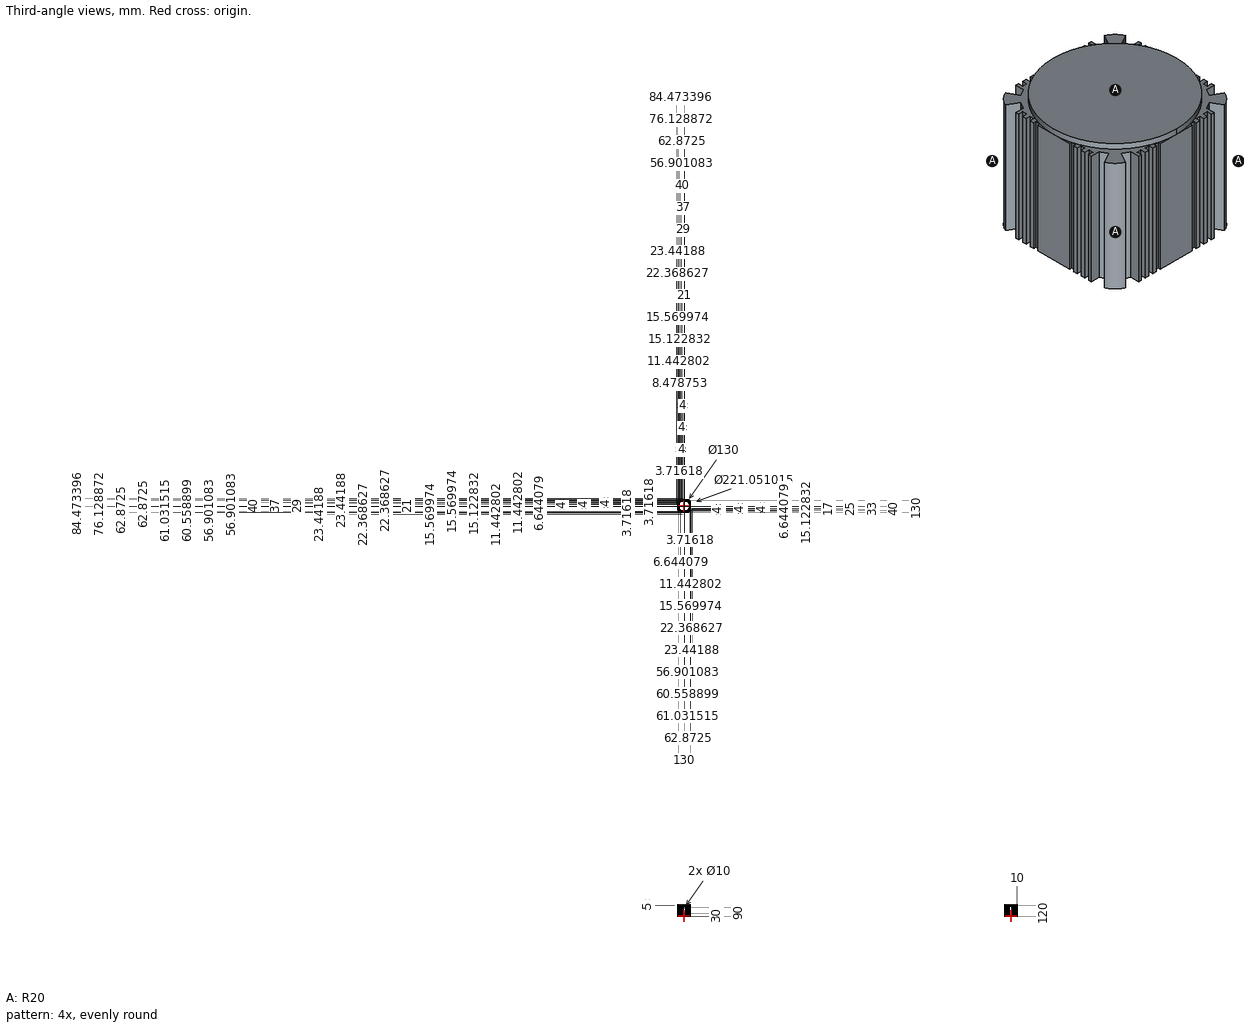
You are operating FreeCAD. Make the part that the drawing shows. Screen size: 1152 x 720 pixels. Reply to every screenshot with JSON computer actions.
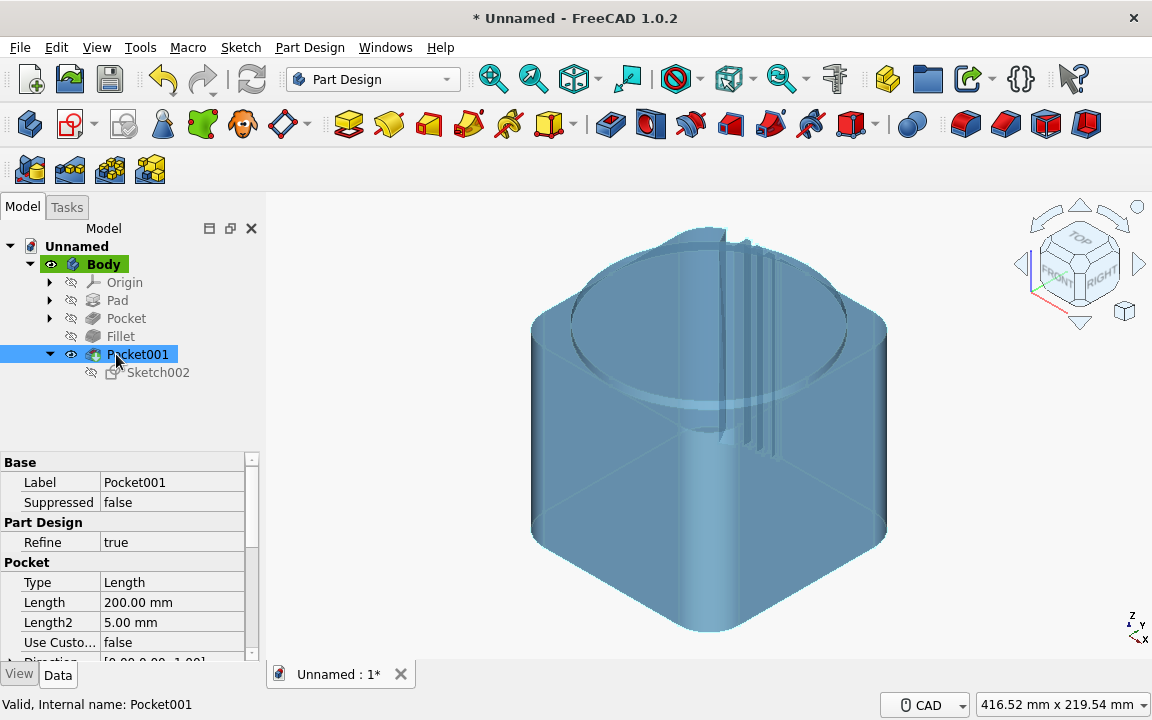
{"action": "left_click", "coordinate": [30, 170]}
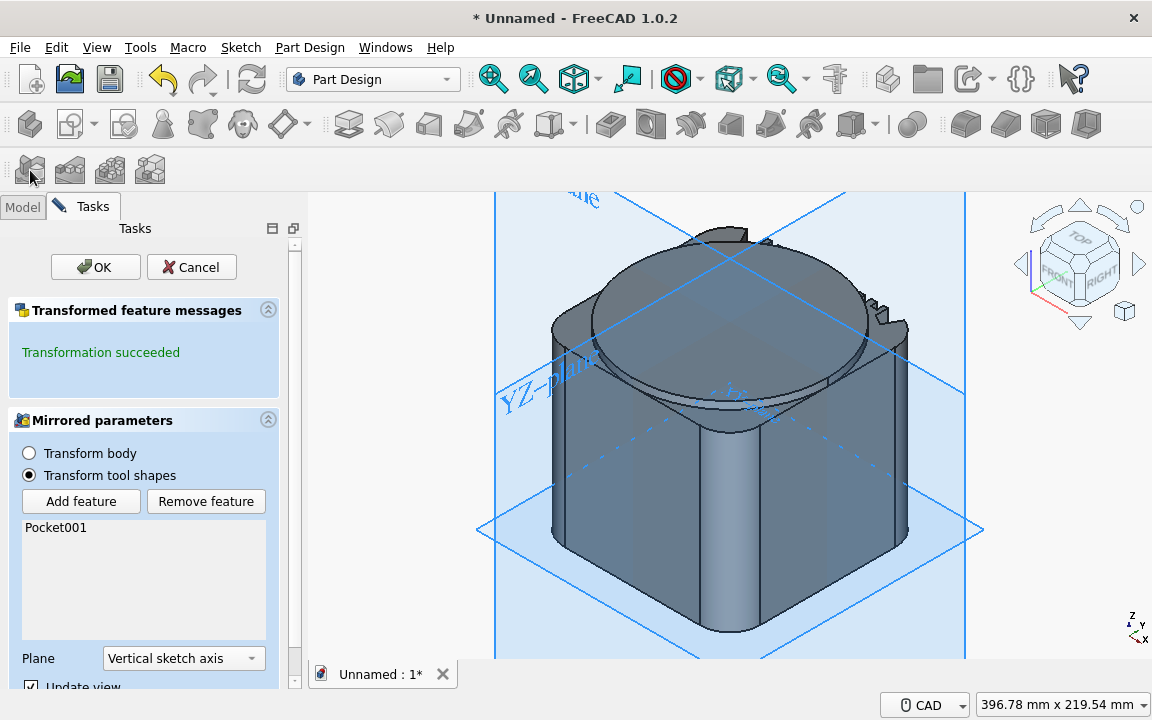
{"action": "left_click", "coordinate": [184, 658]}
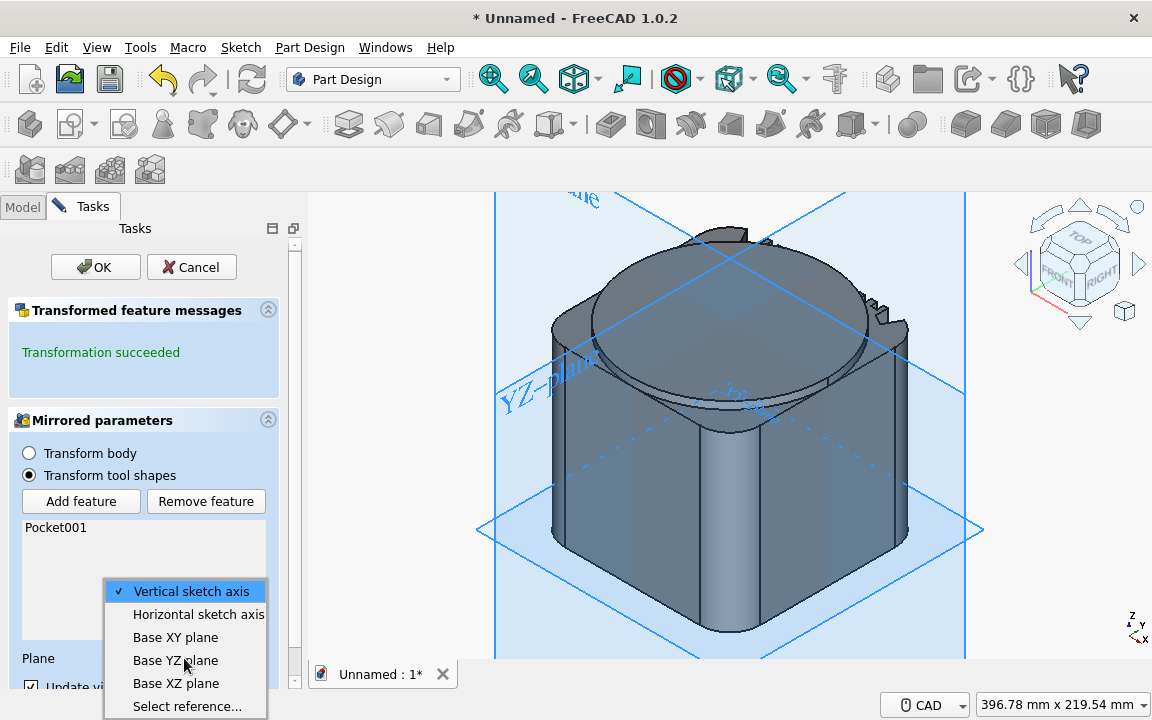
{"action": "left_click", "coordinate": [184, 660]}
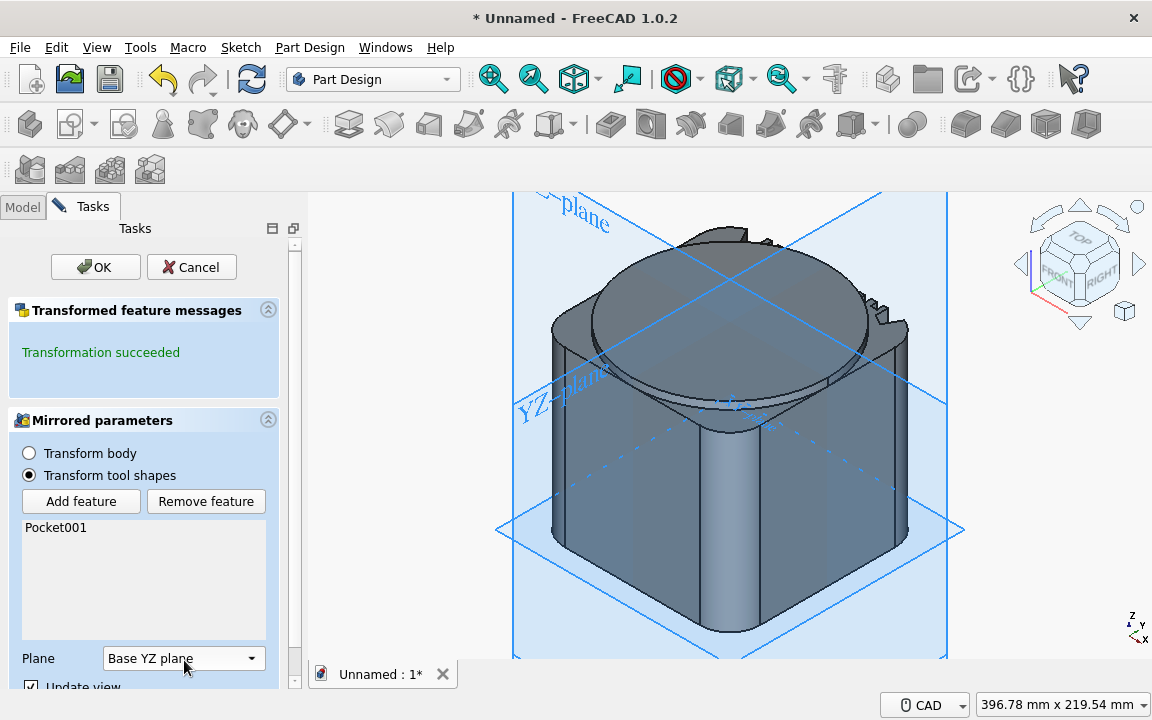
{"action": "left_click", "coordinate": [96, 267]}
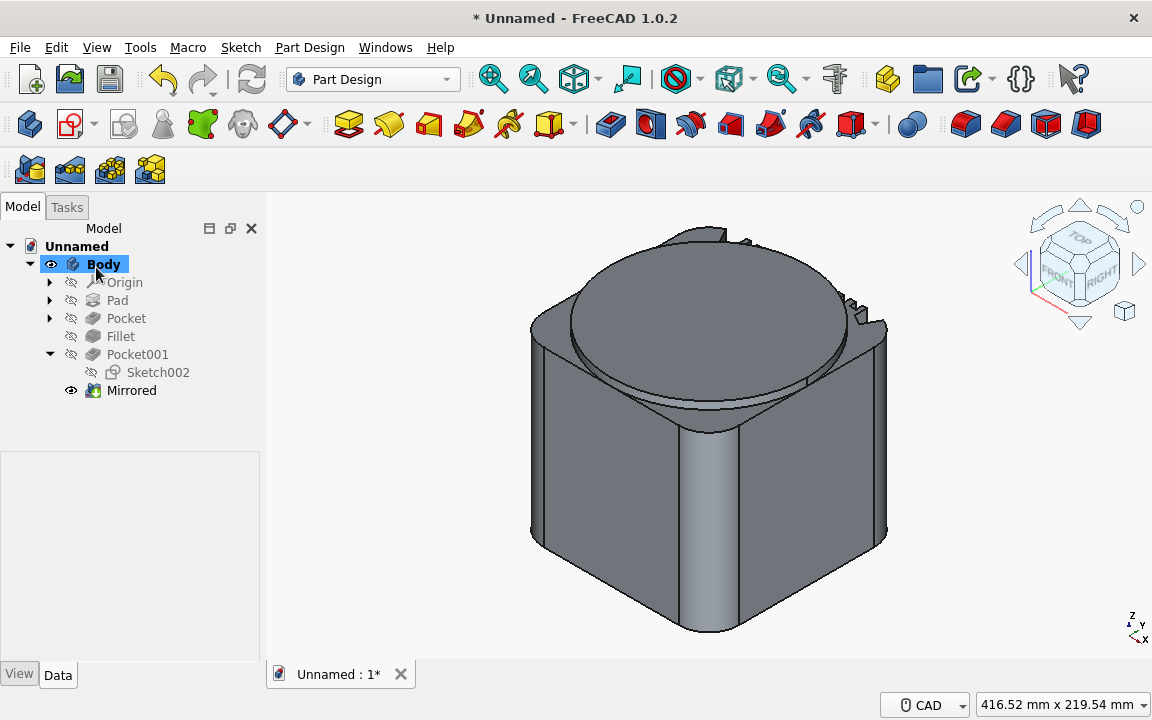
{"action": "left_click", "coordinate": [116, 354]}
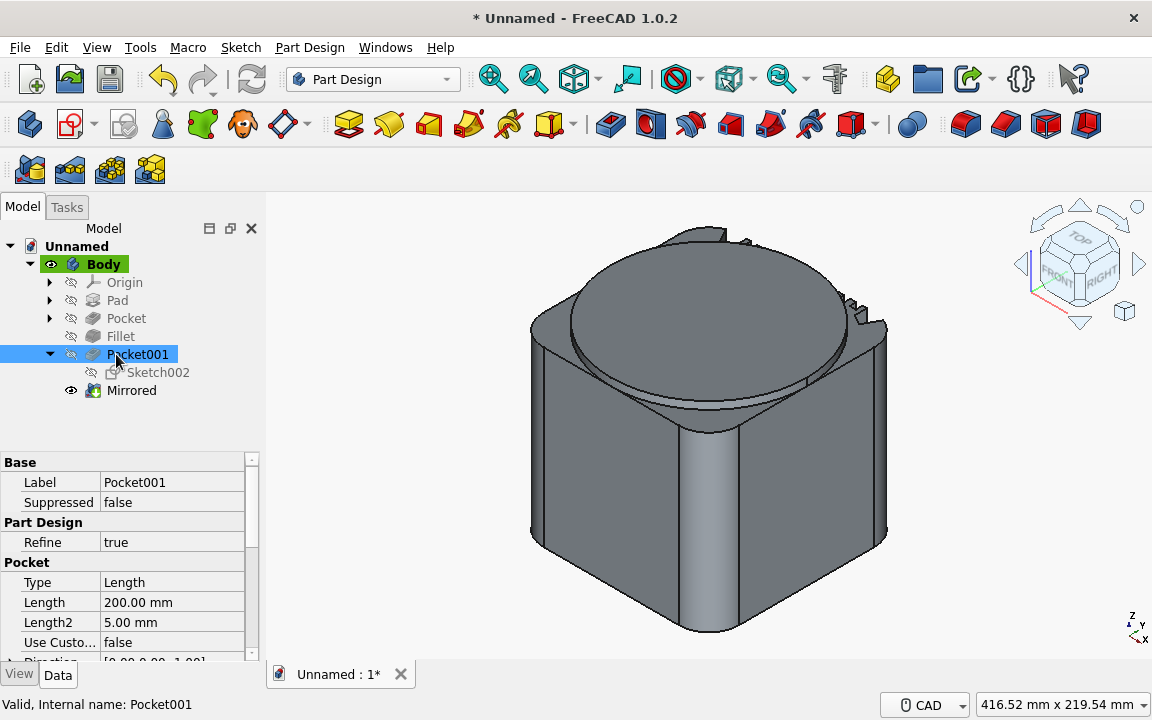
{"action": "left_click", "coordinate": [110, 170]}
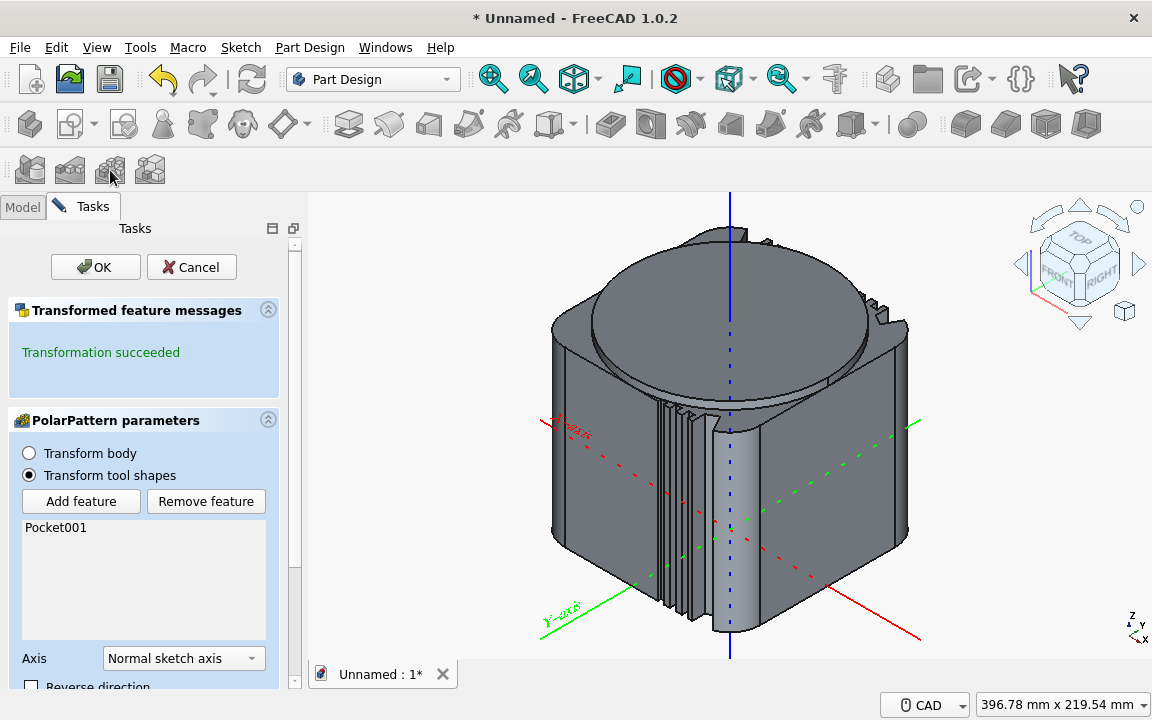
{"action": "left_click", "coordinate": [184, 658]}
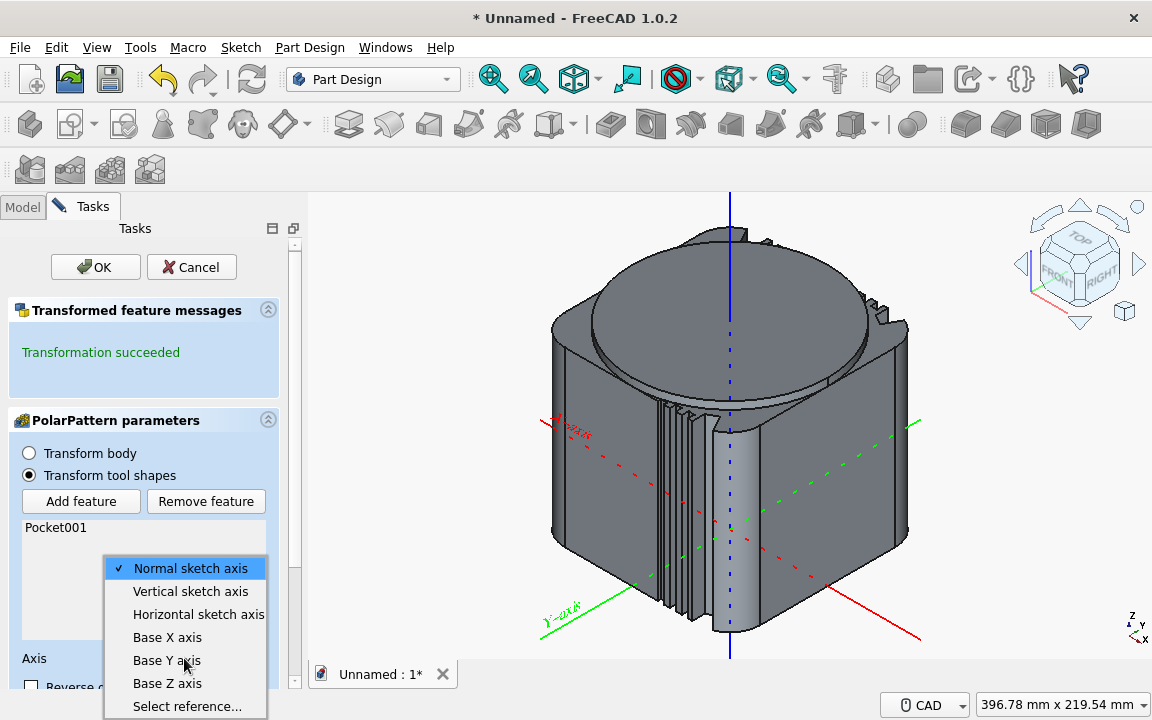
{"action": "left_click", "coordinate": [184, 684]}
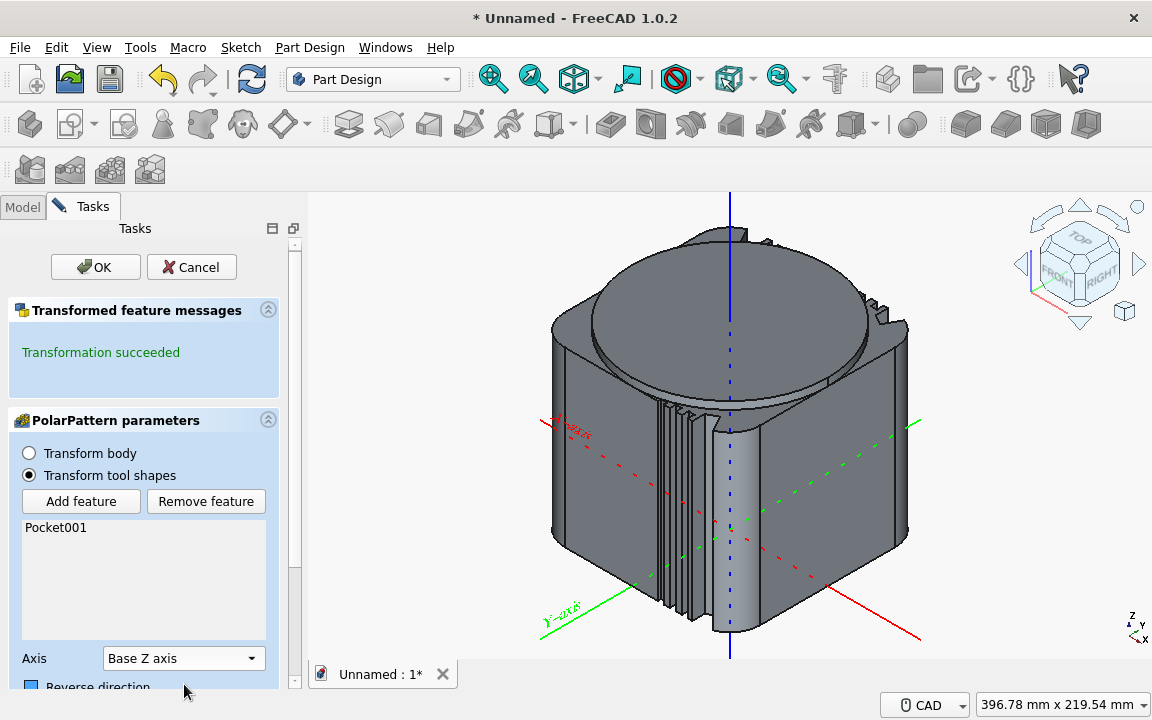
{"action": "scroll", "coordinate": [295, 463], "scroll_direction": "down", "scroll_amount": 3}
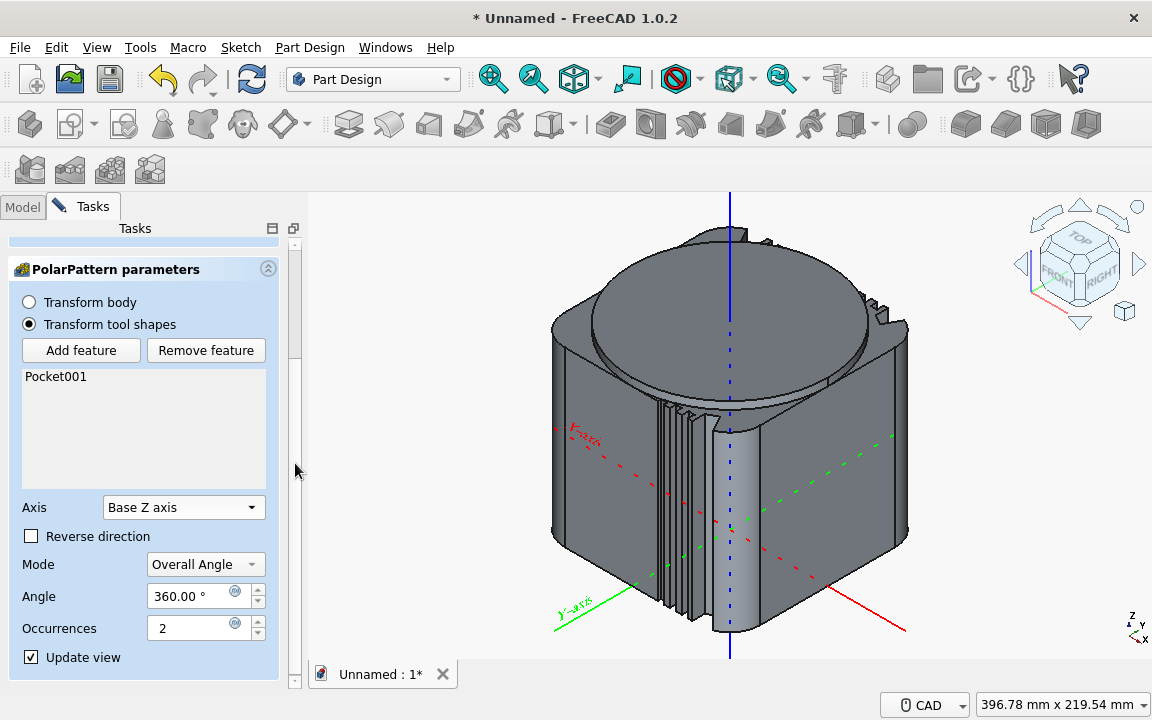
{"action": "triple_click", "coordinate": [198, 628]}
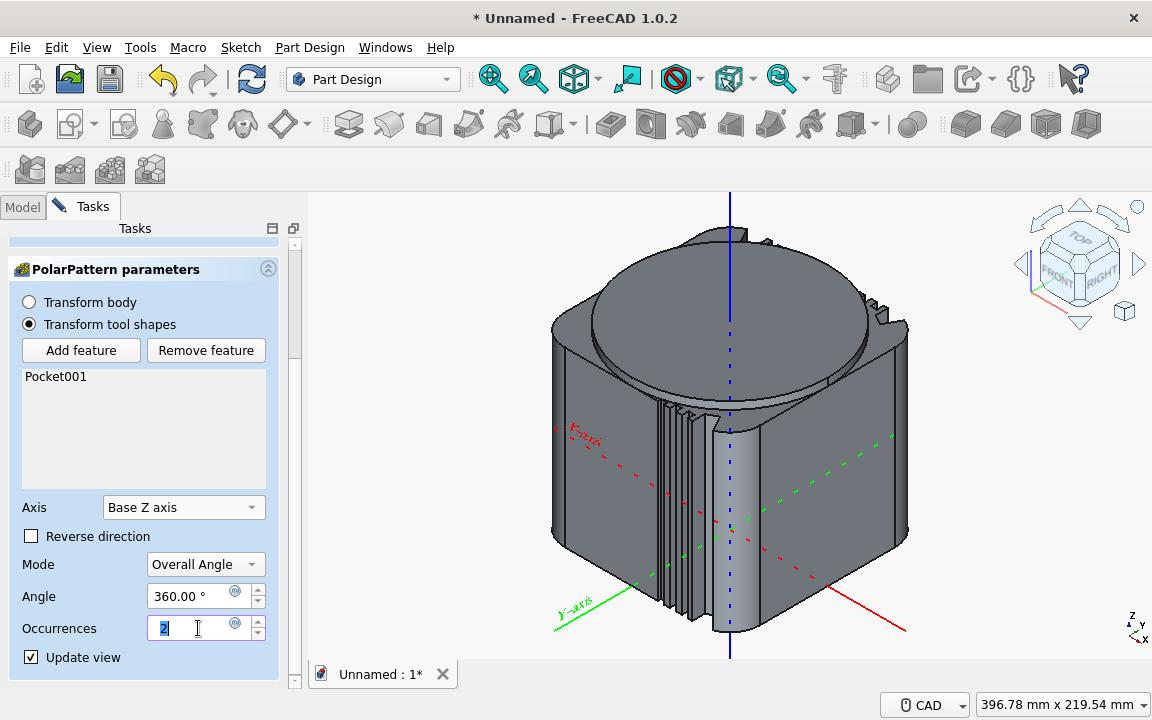
{"action": "type", "text": "4"}
{"action": "key", "text": "Tab"}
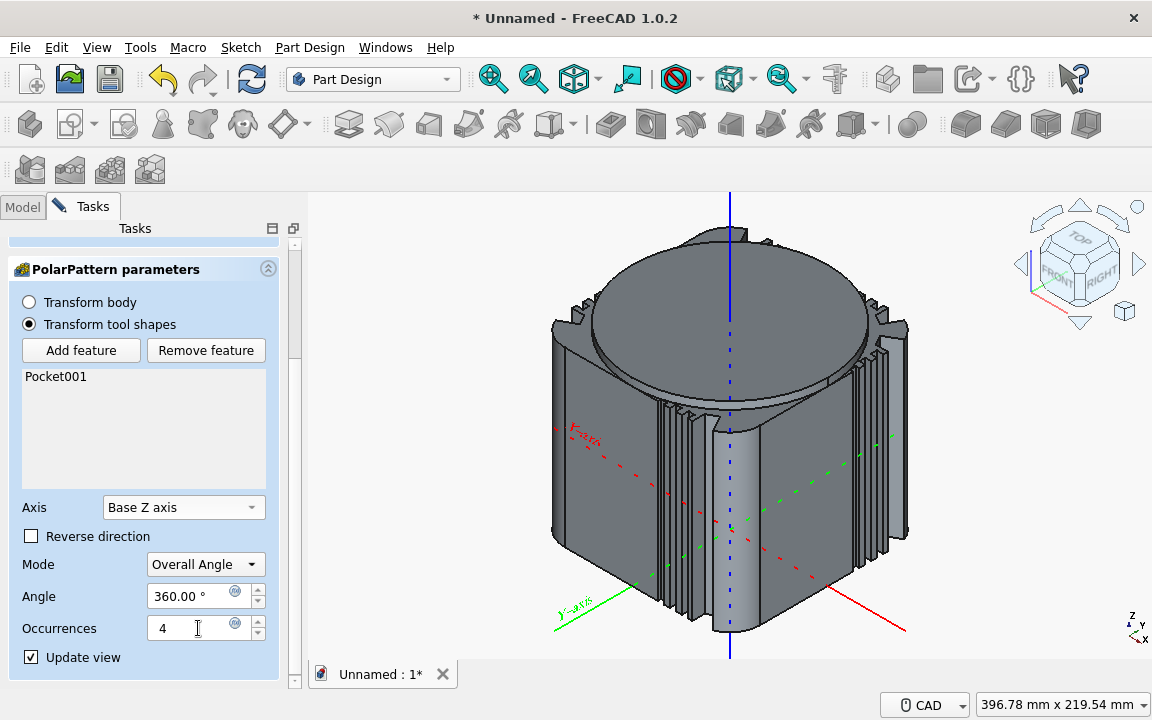
{"action": "scroll", "coordinate": [295, 463], "scroll_direction": "up", "scroll_amount": 4}